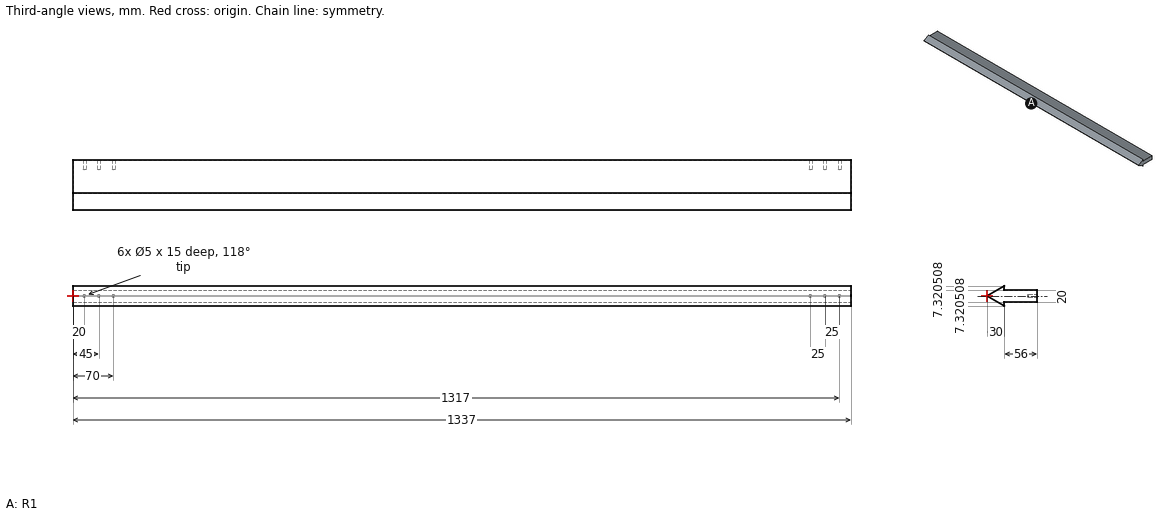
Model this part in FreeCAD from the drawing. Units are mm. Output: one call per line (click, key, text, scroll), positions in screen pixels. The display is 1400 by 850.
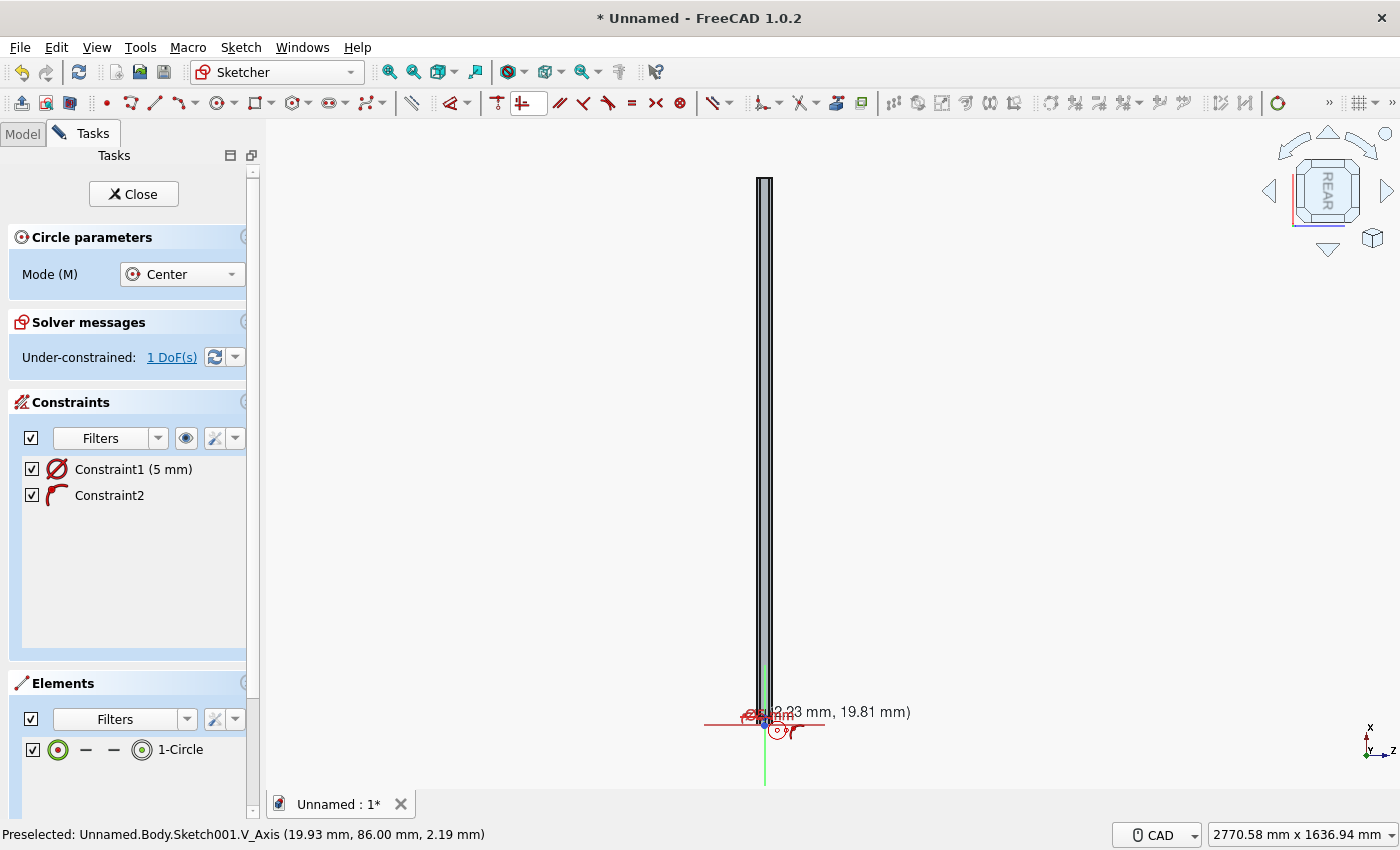
scroll(765, 707, up, 3)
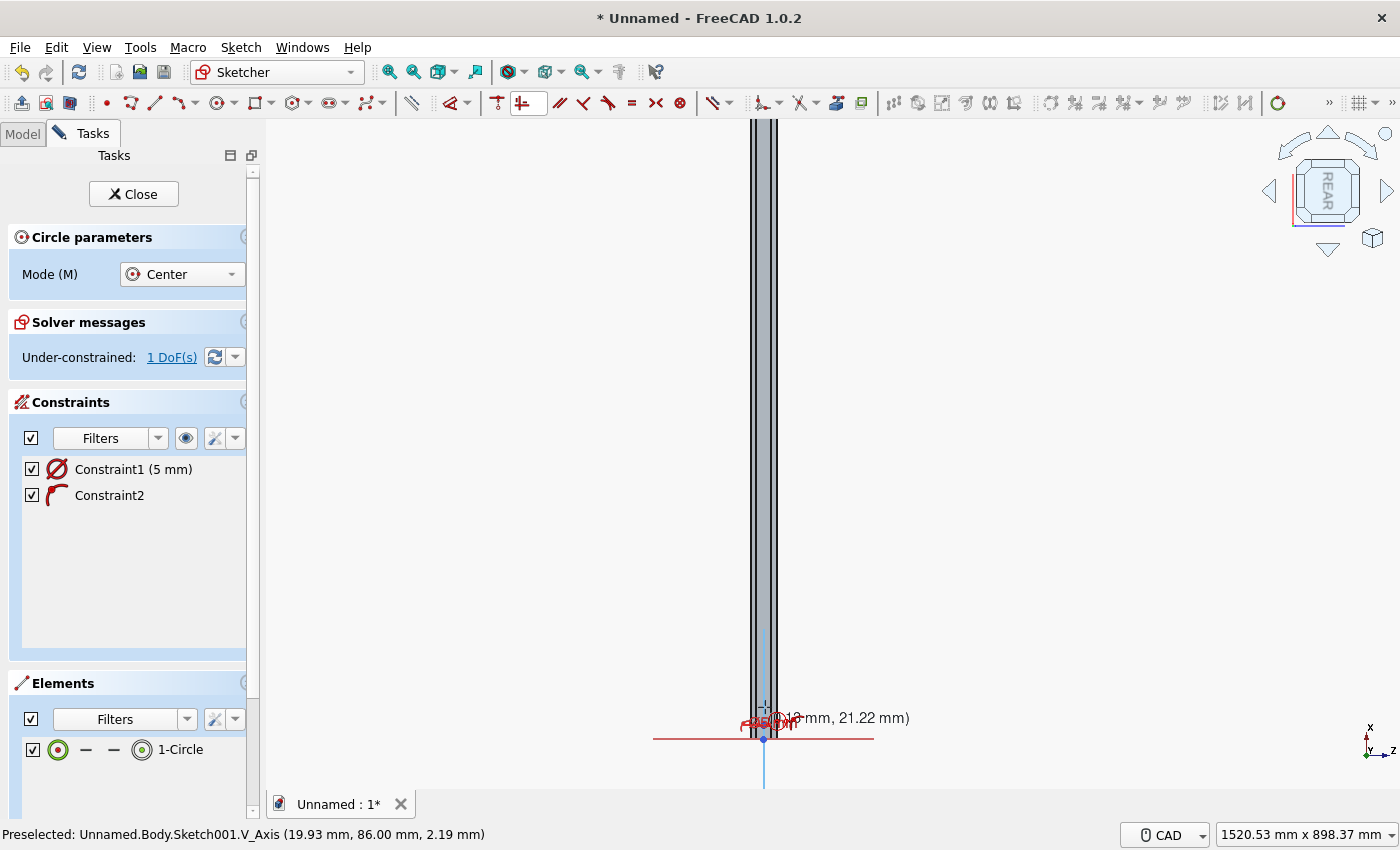
click(764, 706)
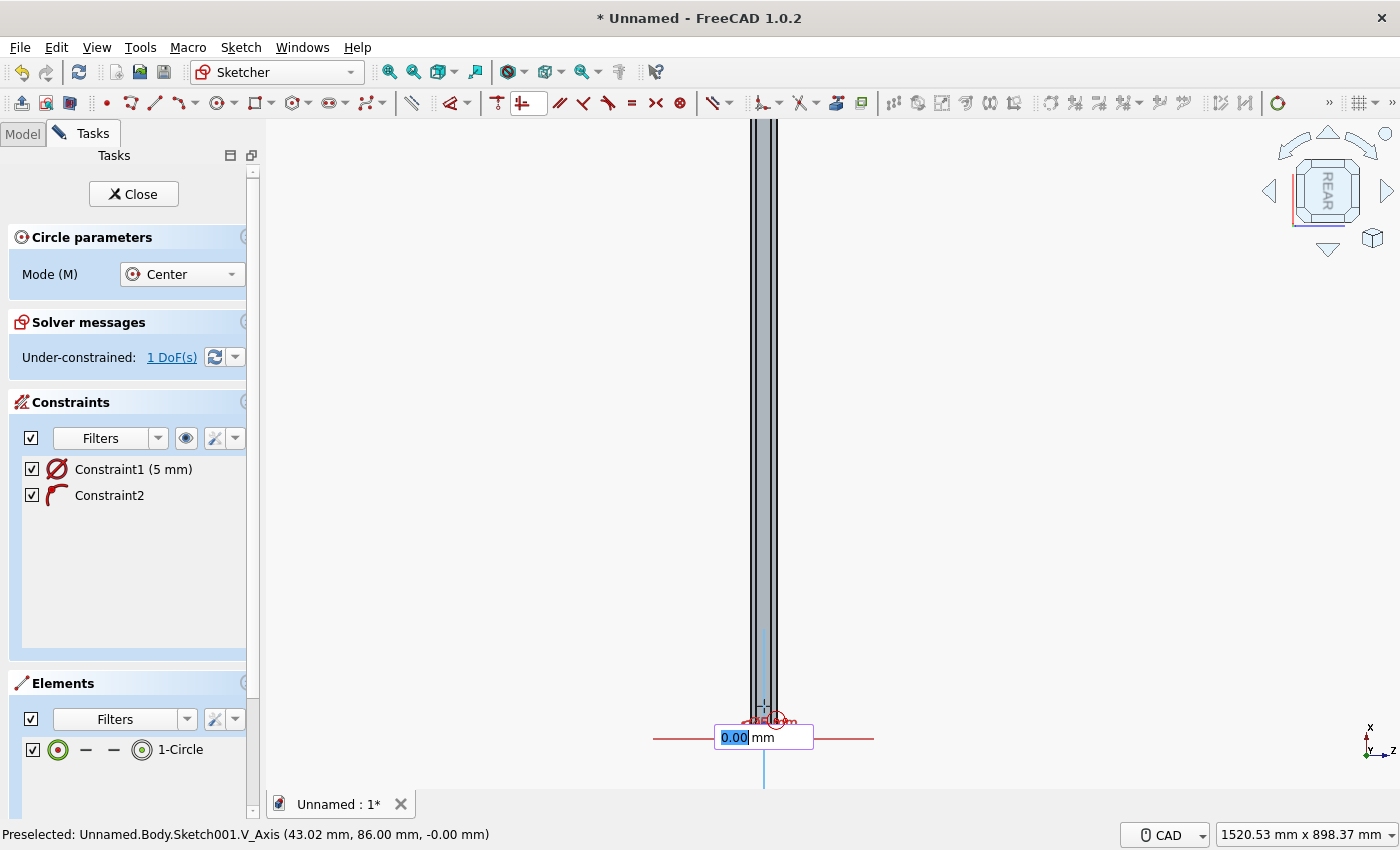
scroll(765, 705, up, 12)
move(766, 695)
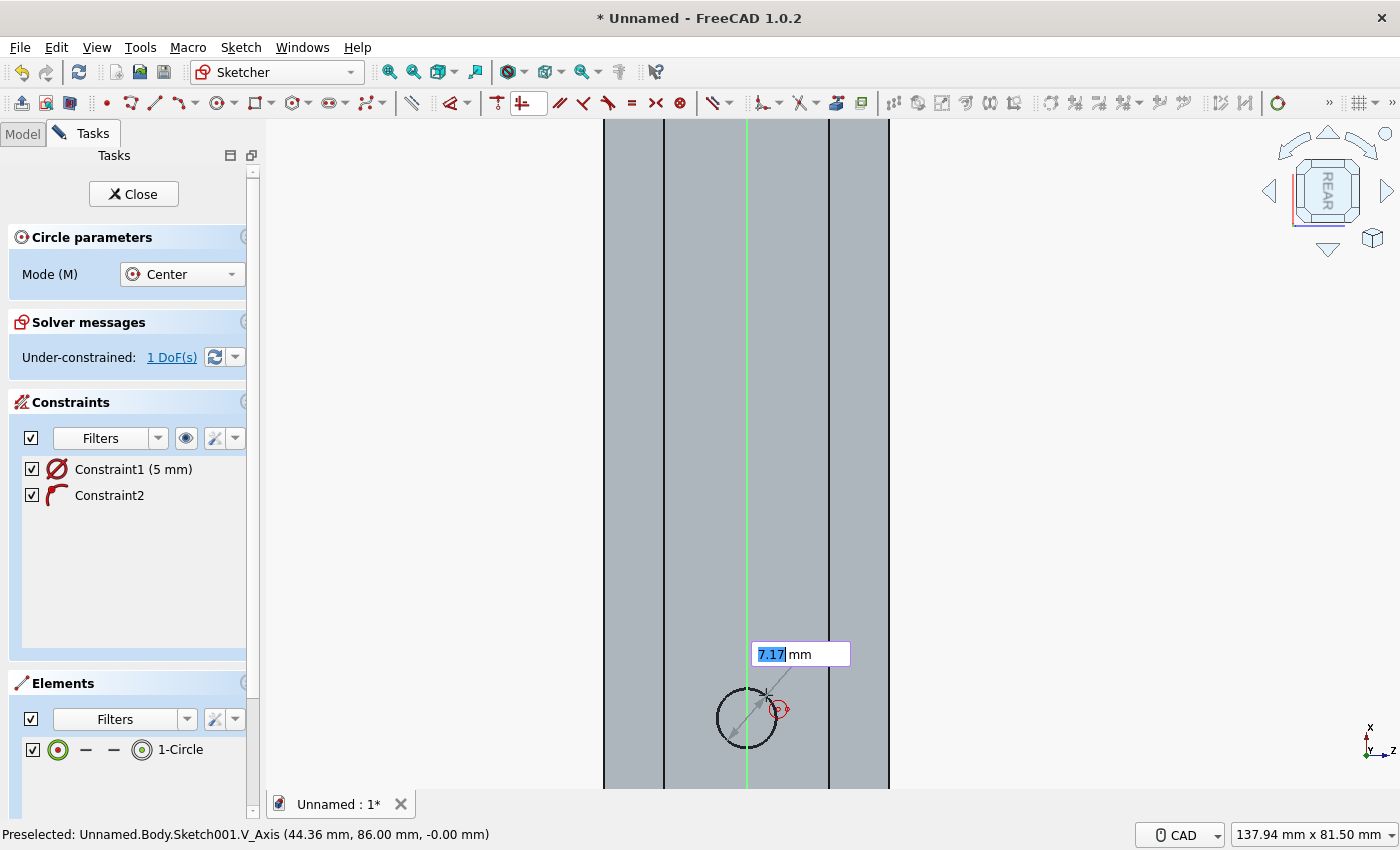
text(5)
key(Return)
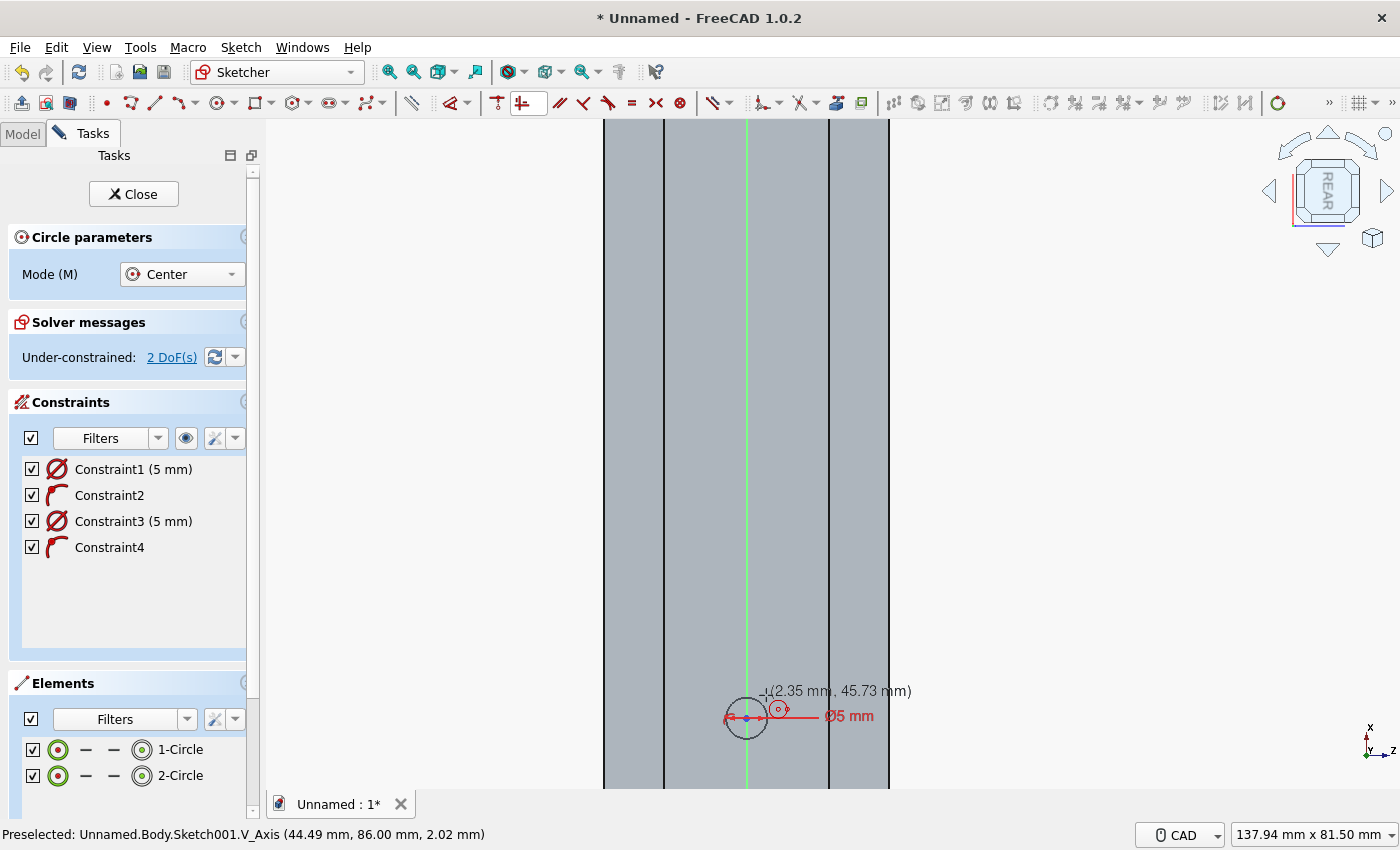
scroll(765, 706, down, 15)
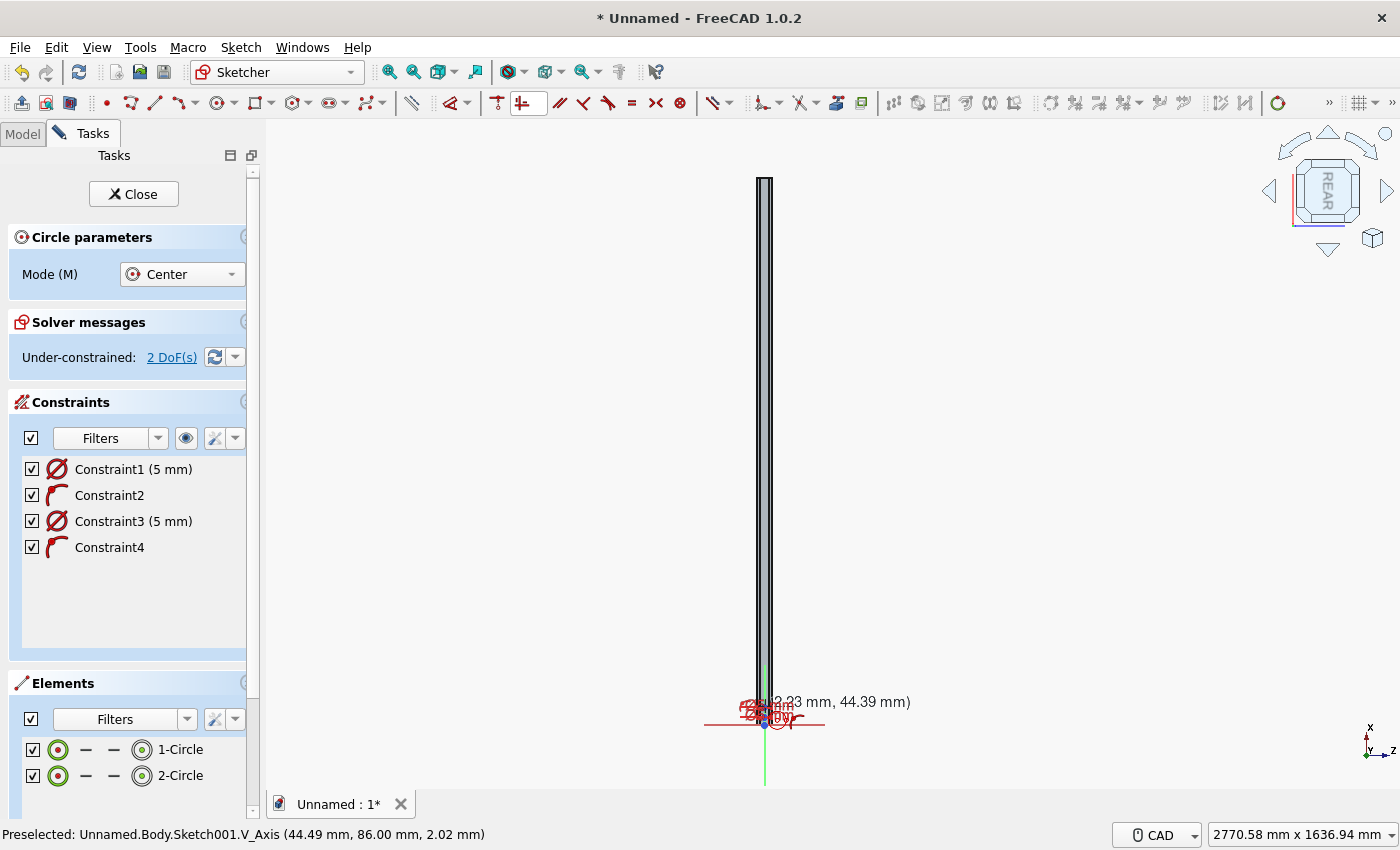
scroll(765, 696, up, 3)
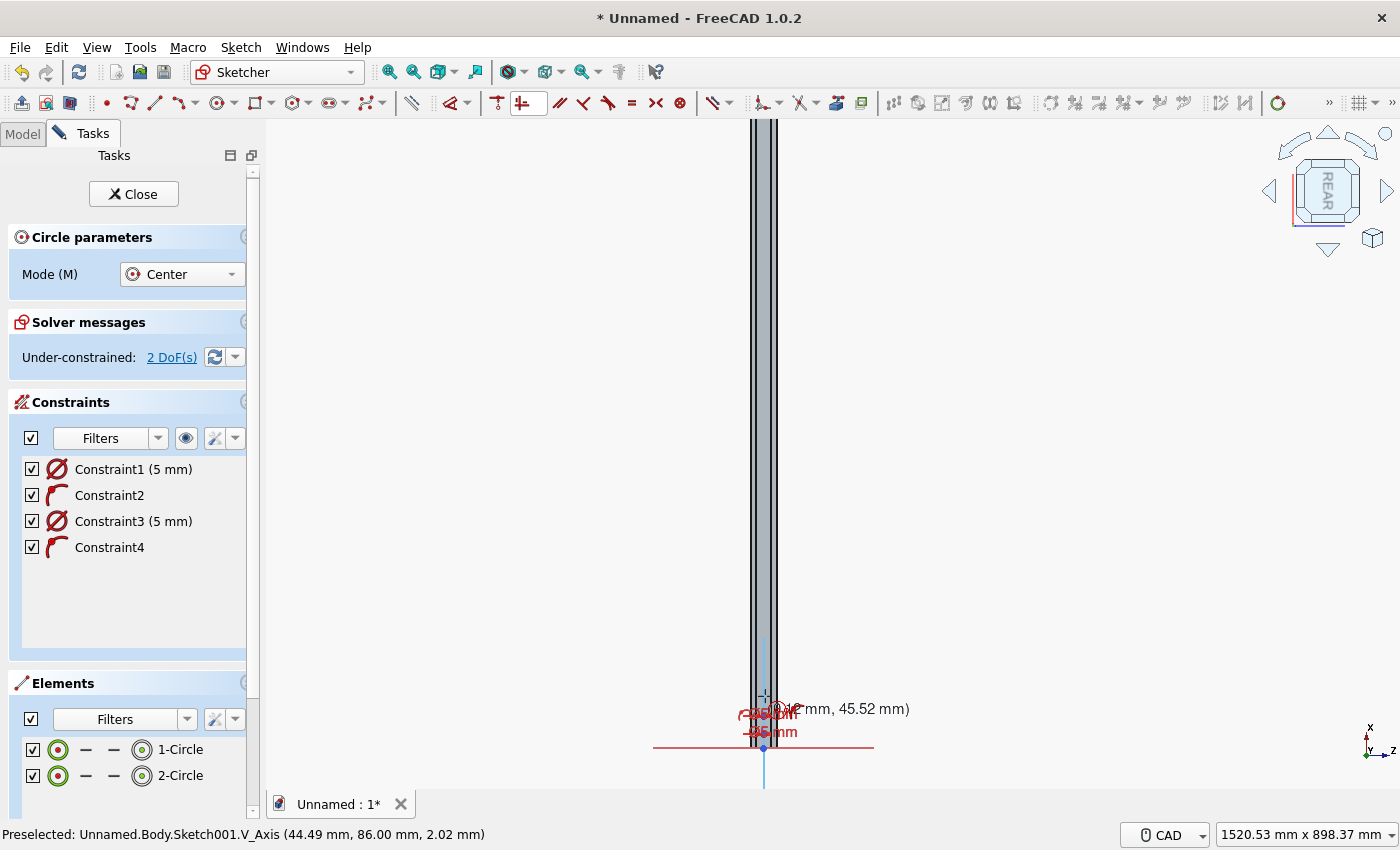
click(764, 696)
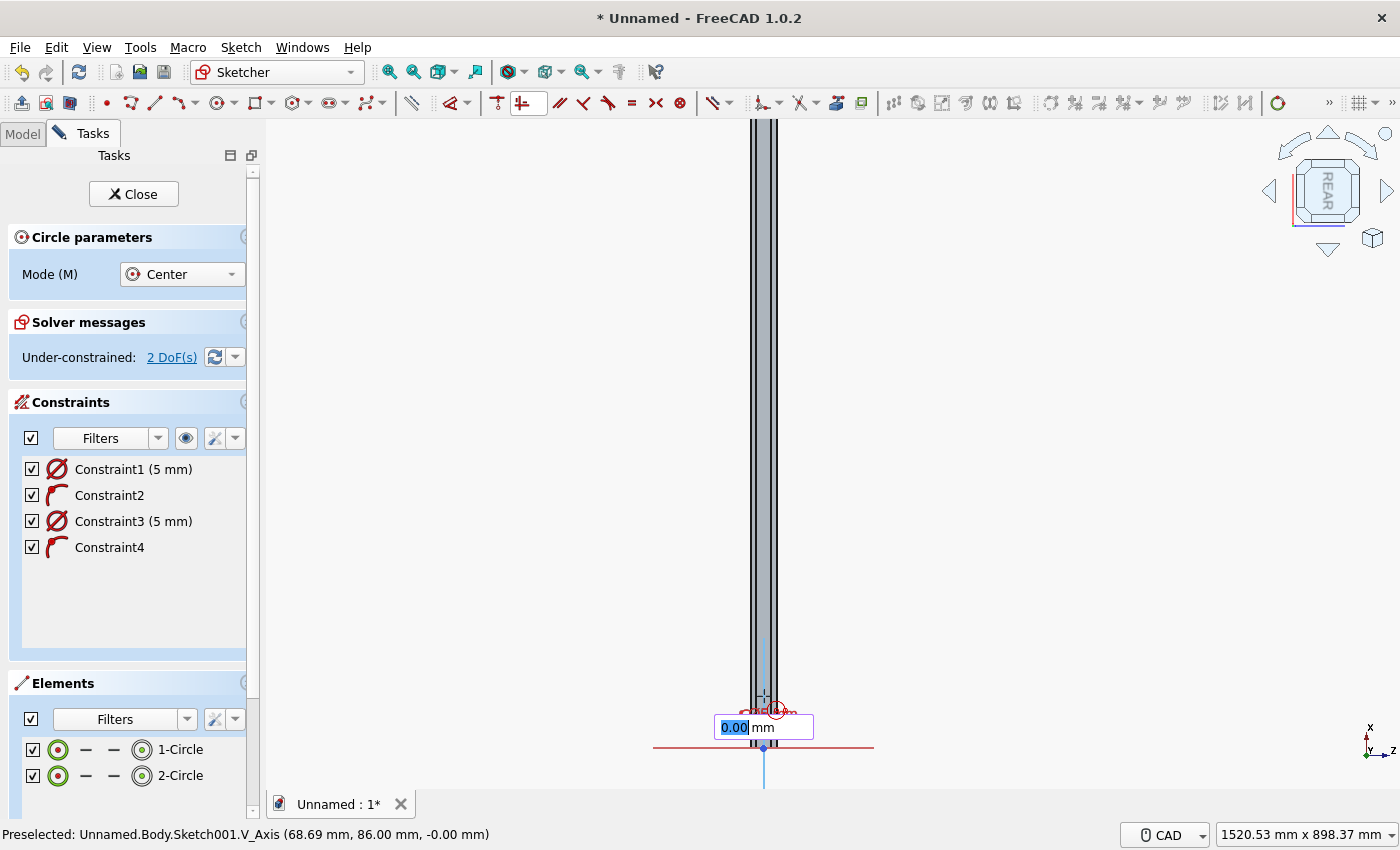
scroll(765, 695, up, 12)
move(766, 691)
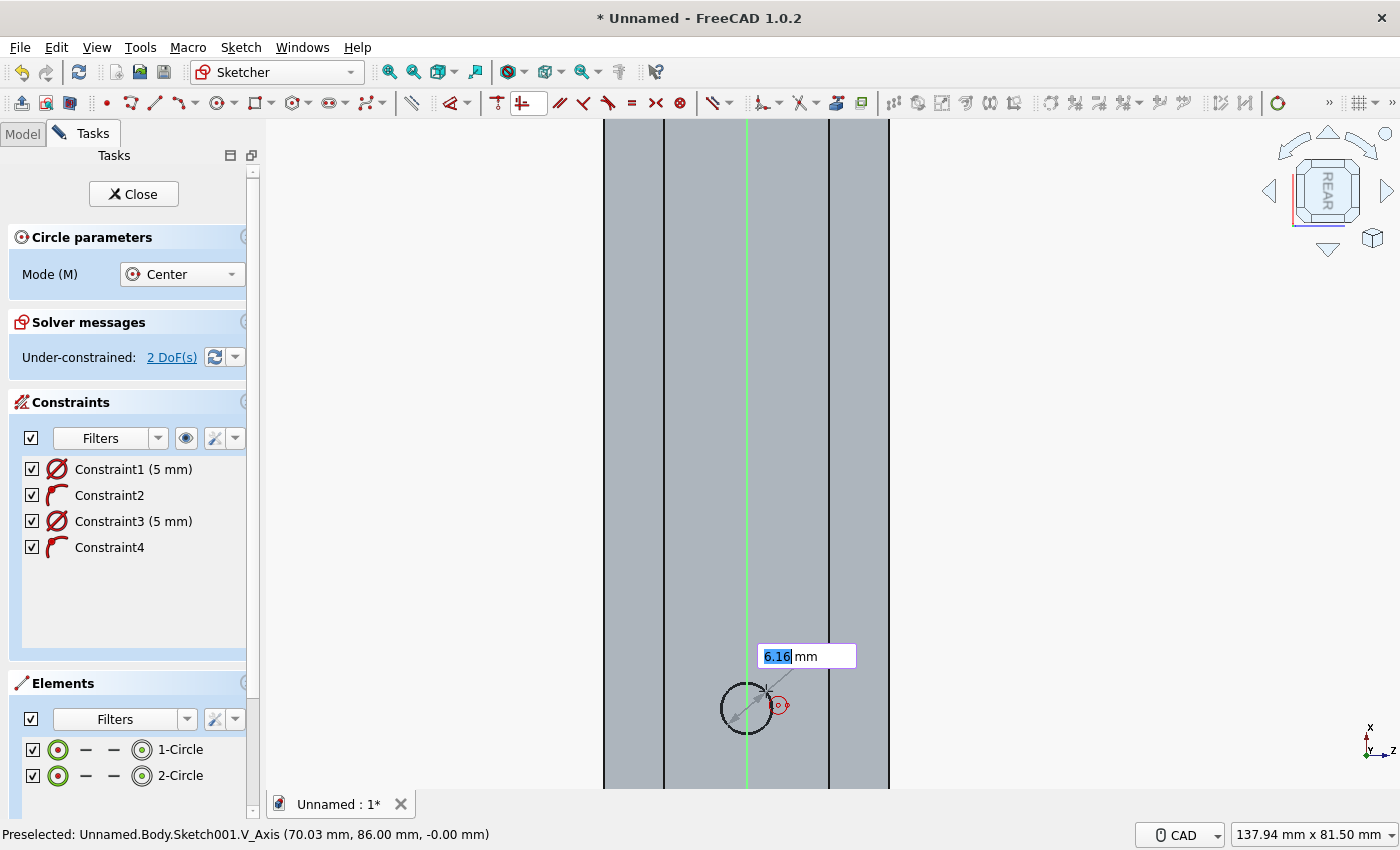
text(5)
key(Return)